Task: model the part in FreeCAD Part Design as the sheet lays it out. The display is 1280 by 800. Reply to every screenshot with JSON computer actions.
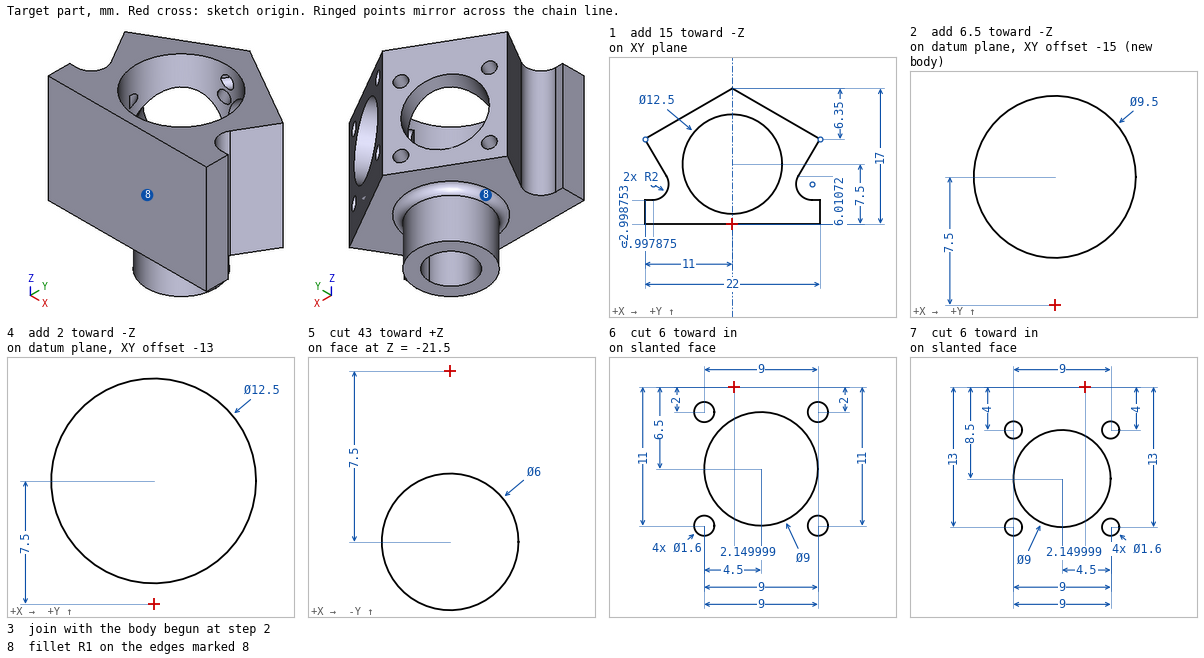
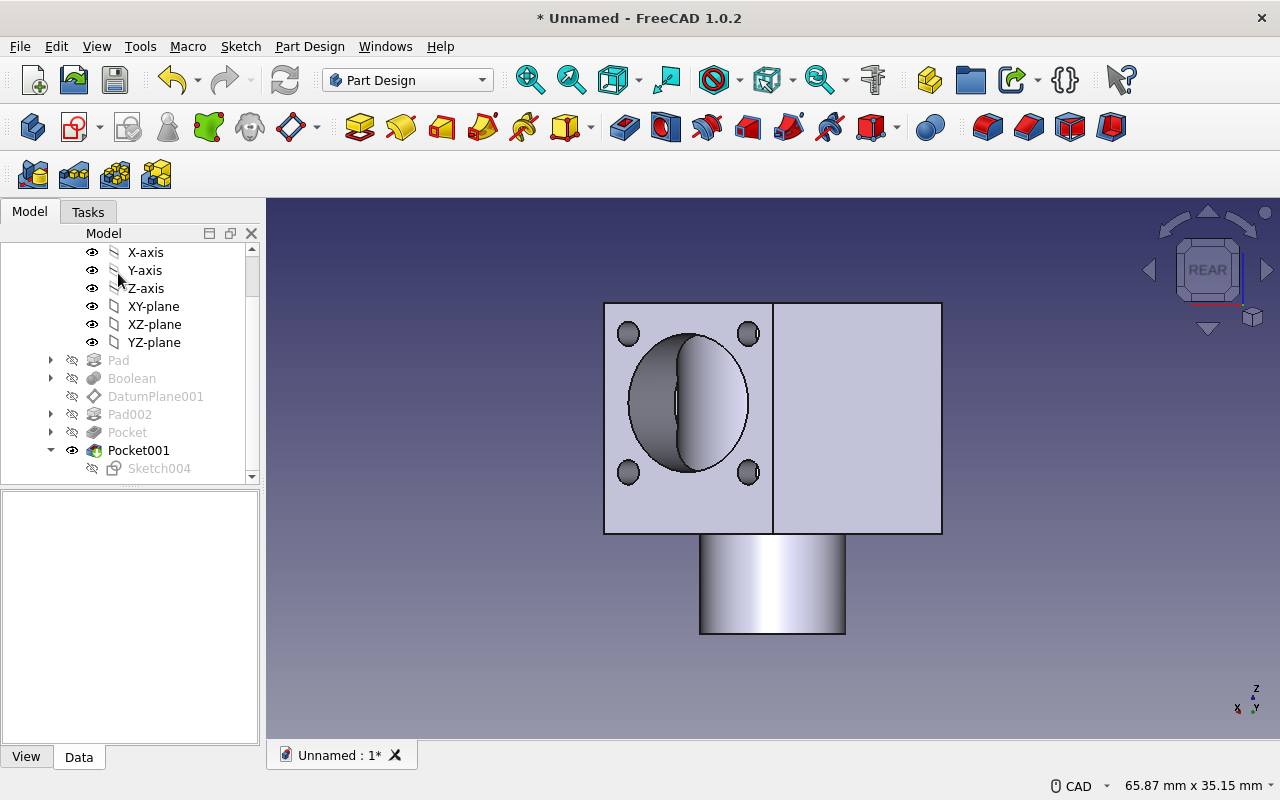
{"action": "left_click", "coordinate": [858, 417]}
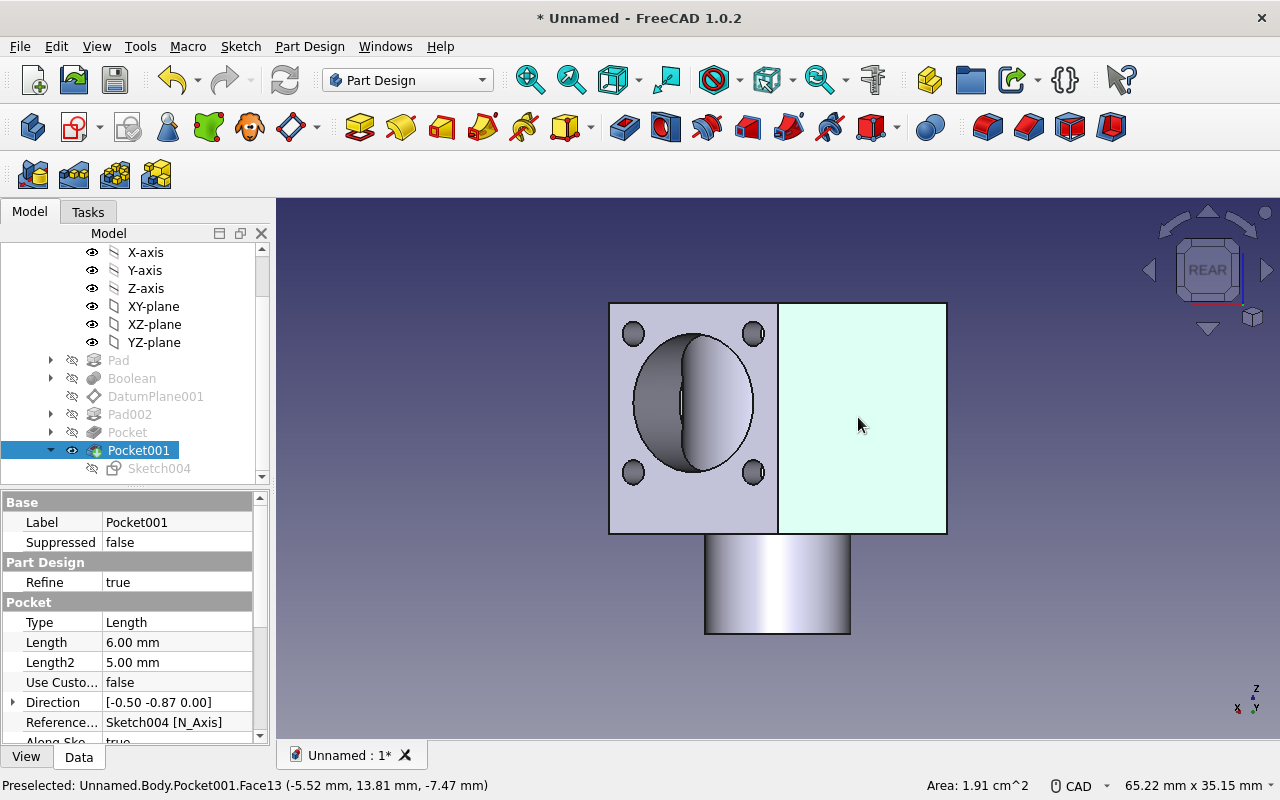
{"action": "left_click", "coordinate": [74, 128]}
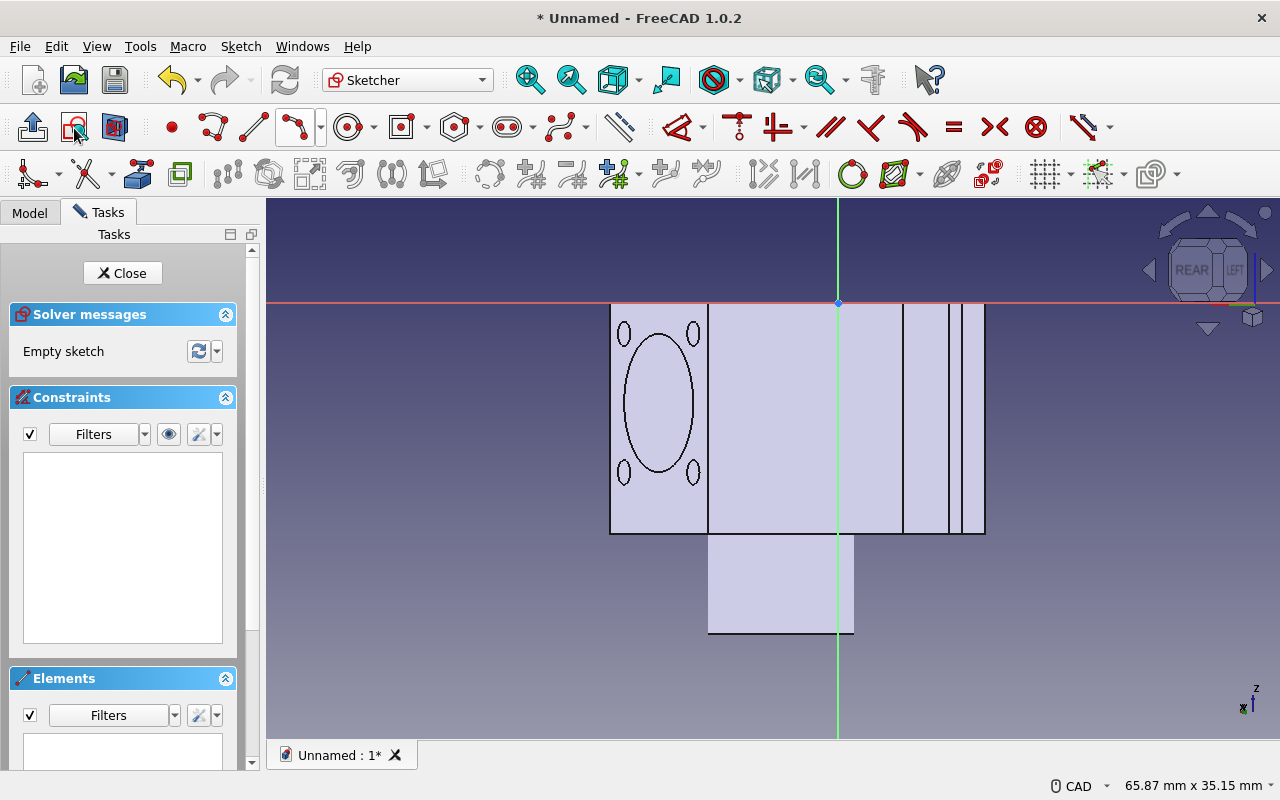
{"action": "left_click", "coordinate": [115, 128]}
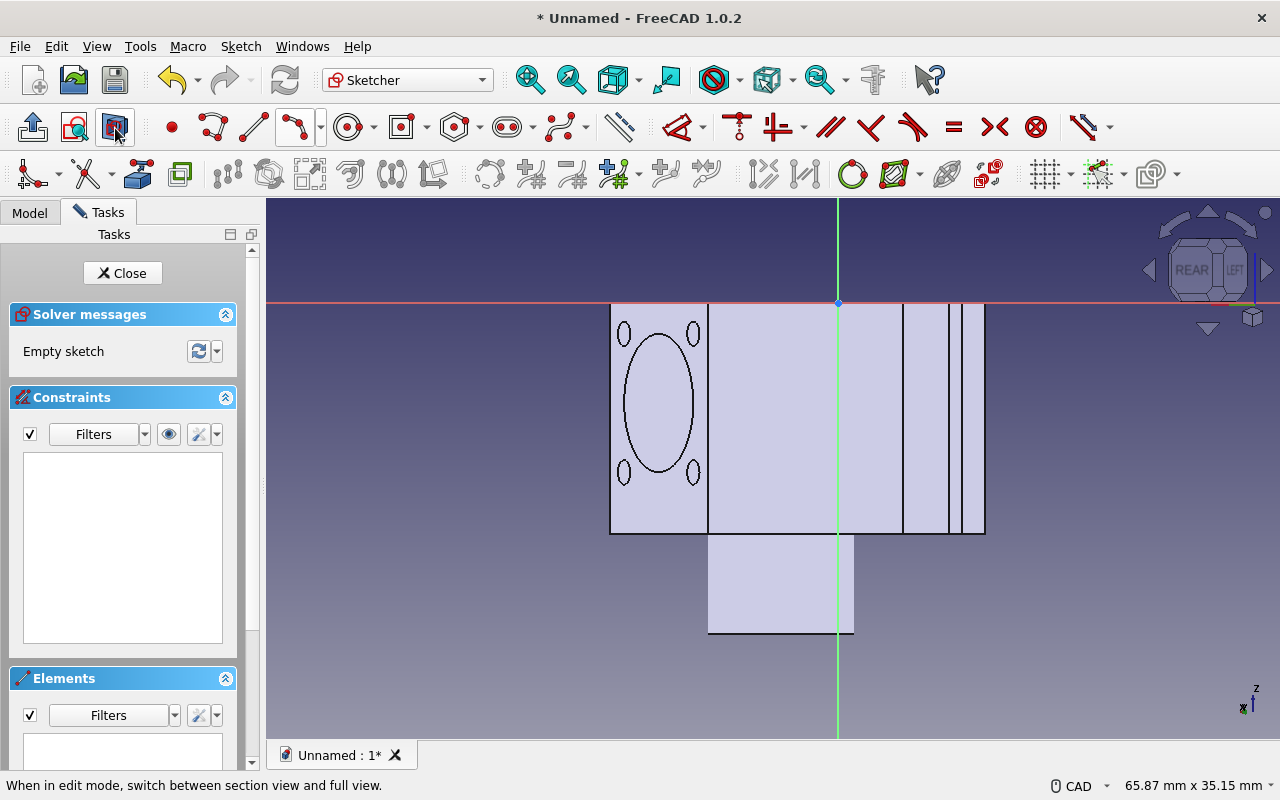
{"action": "scroll", "coordinate": [1010, 289], "scroll_direction": "up", "scroll_amount": 2}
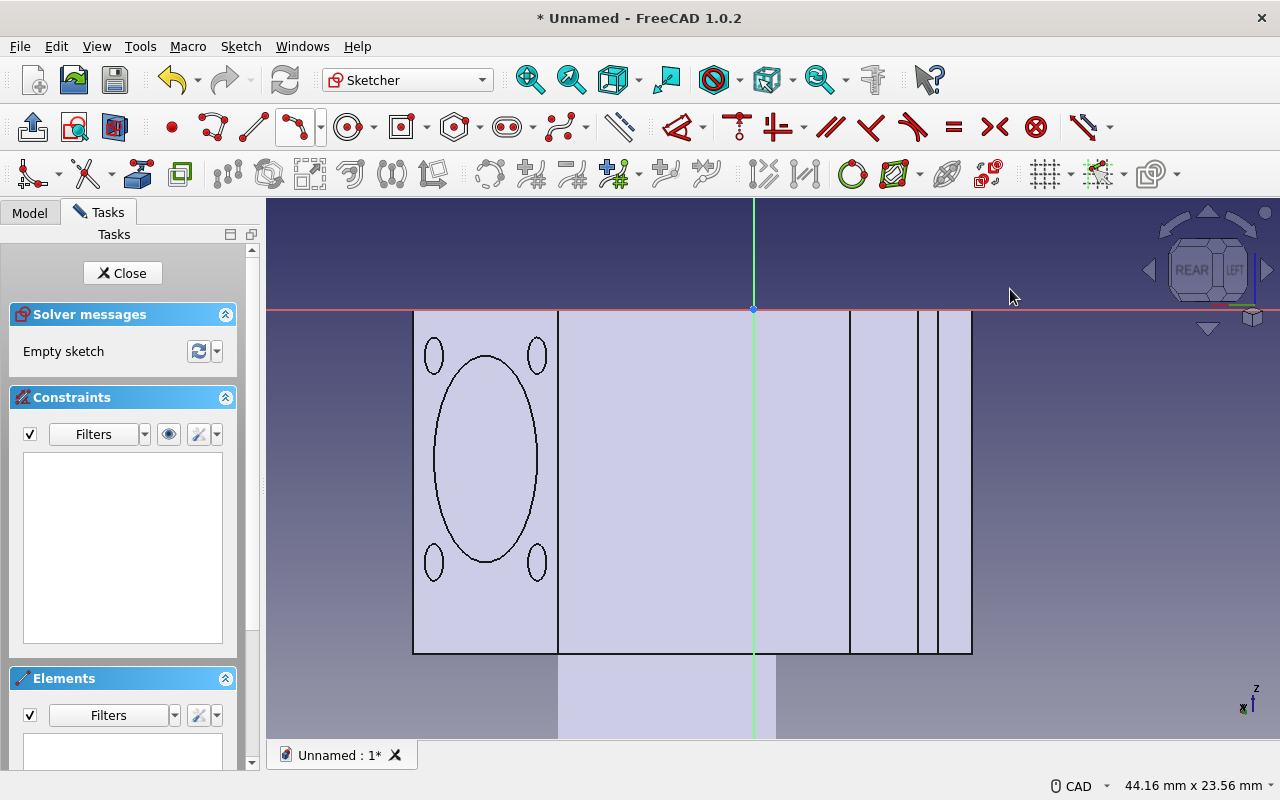
{"action": "left_click", "coordinate": [348, 128]}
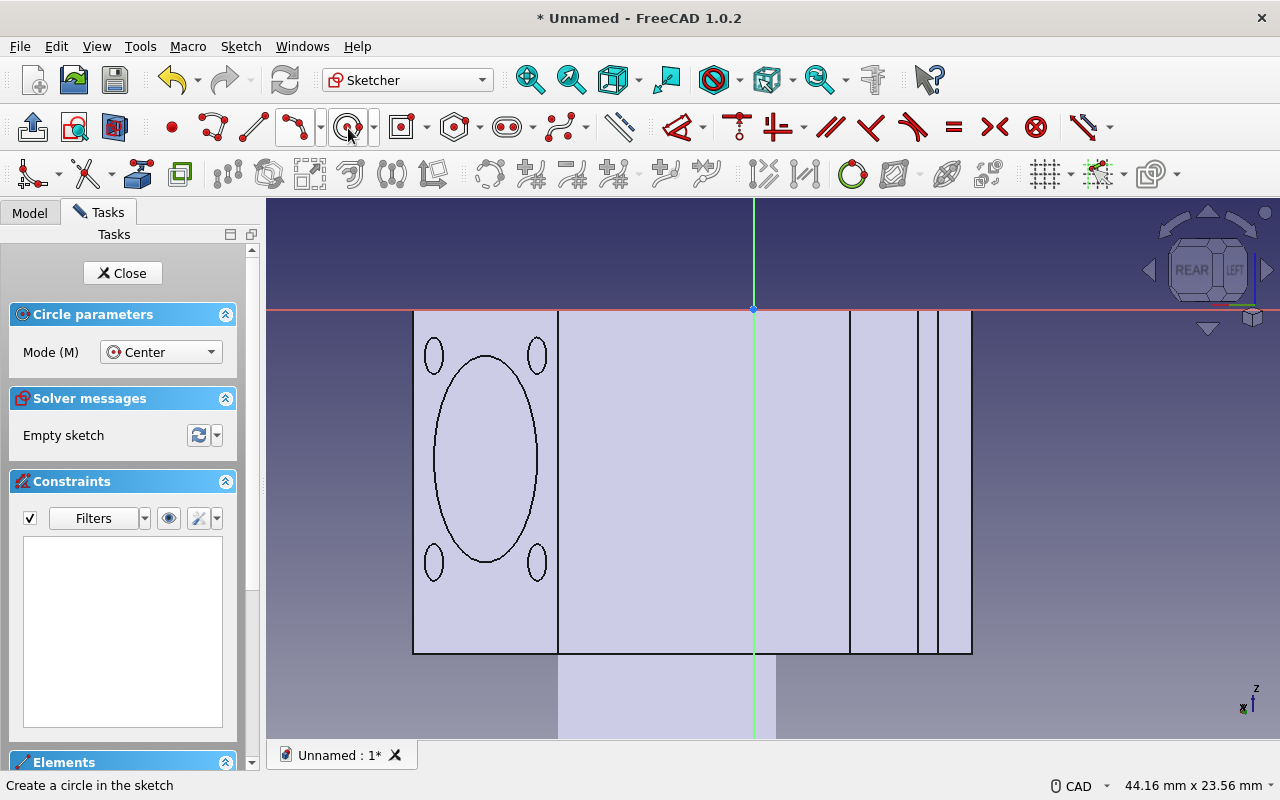
{"action": "left_click", "coordinate": [704, 505]}
{"action": "mouse_move", "coordinate": [777, 432]}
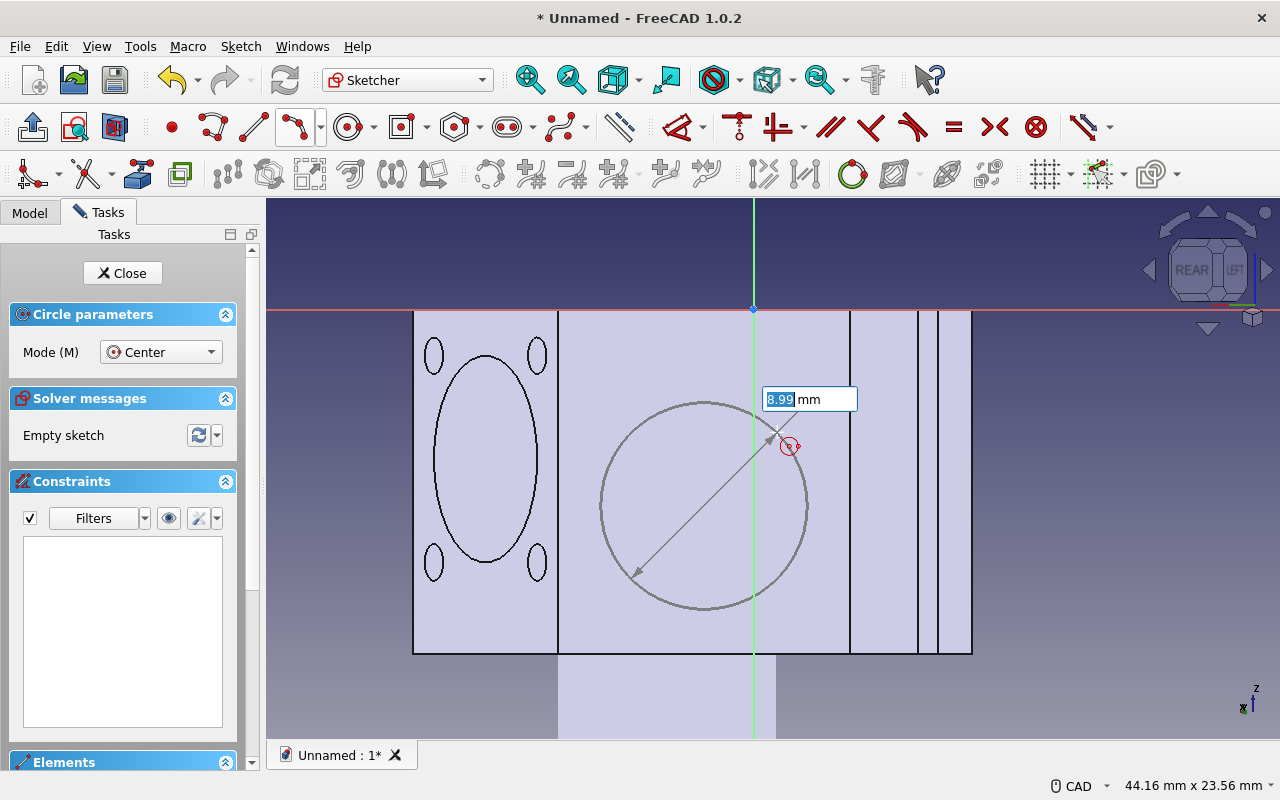
{"action": "type", "text": "9"}
{"action": "key", "text": "Return"}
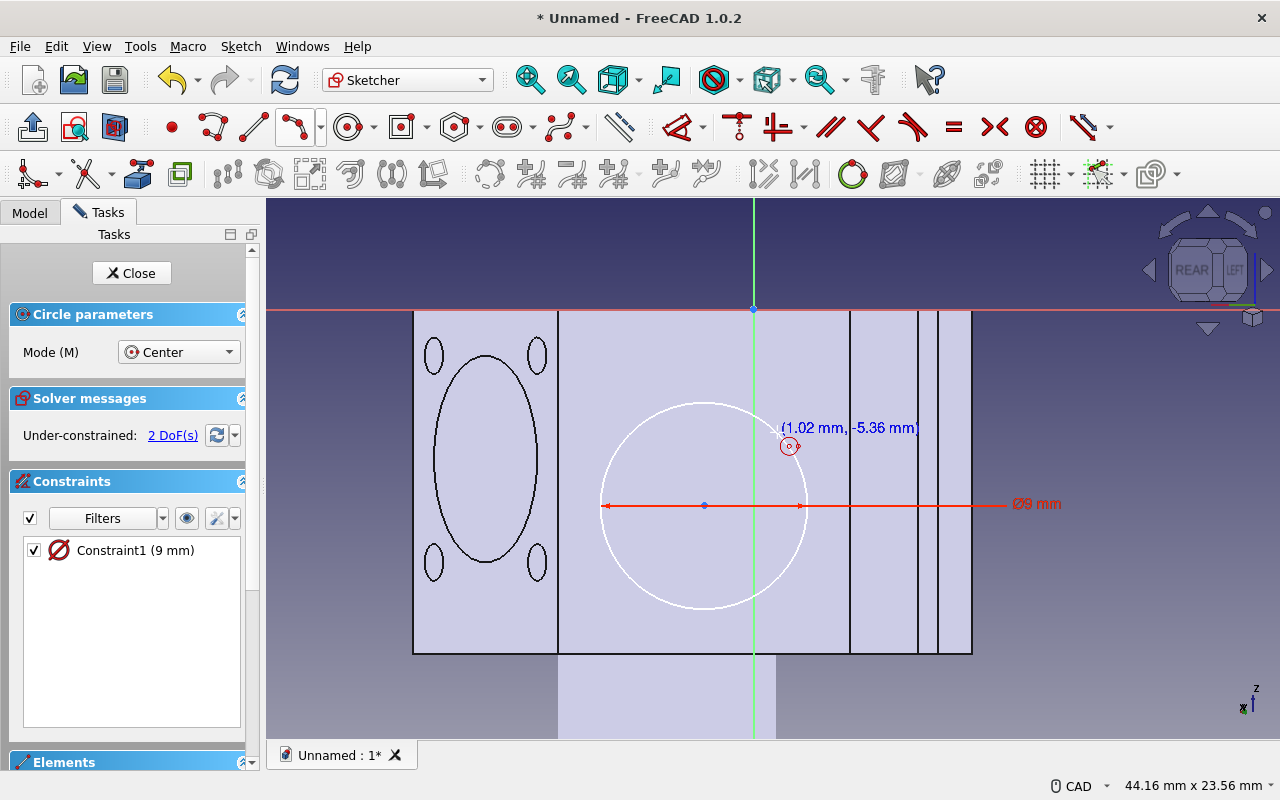
{"action": "scroll", "coordinate": [808, 608], "scroll_direction": "up", "scroll_amount": 2}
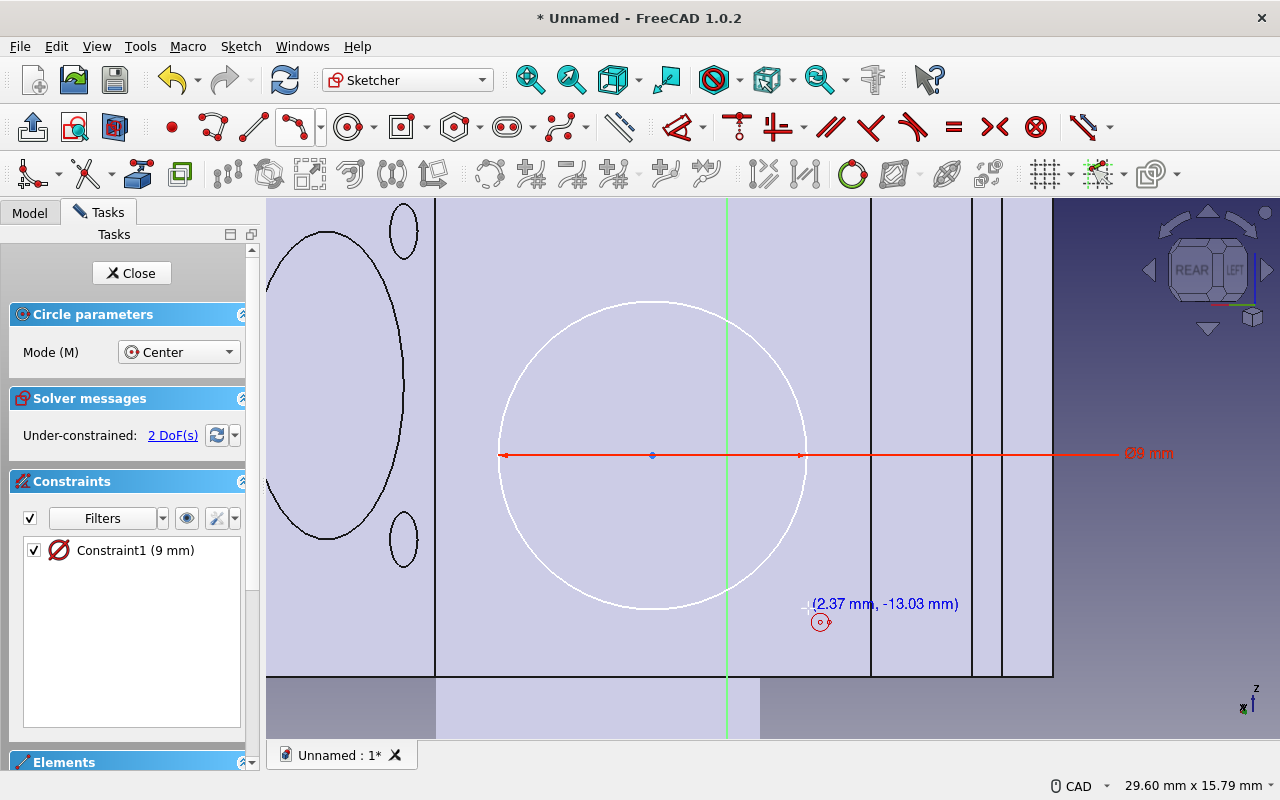
{"action": "left_click", "coordinate": [807, 608]}
{"action": "mouse_move", "coordinate": [827, 589]}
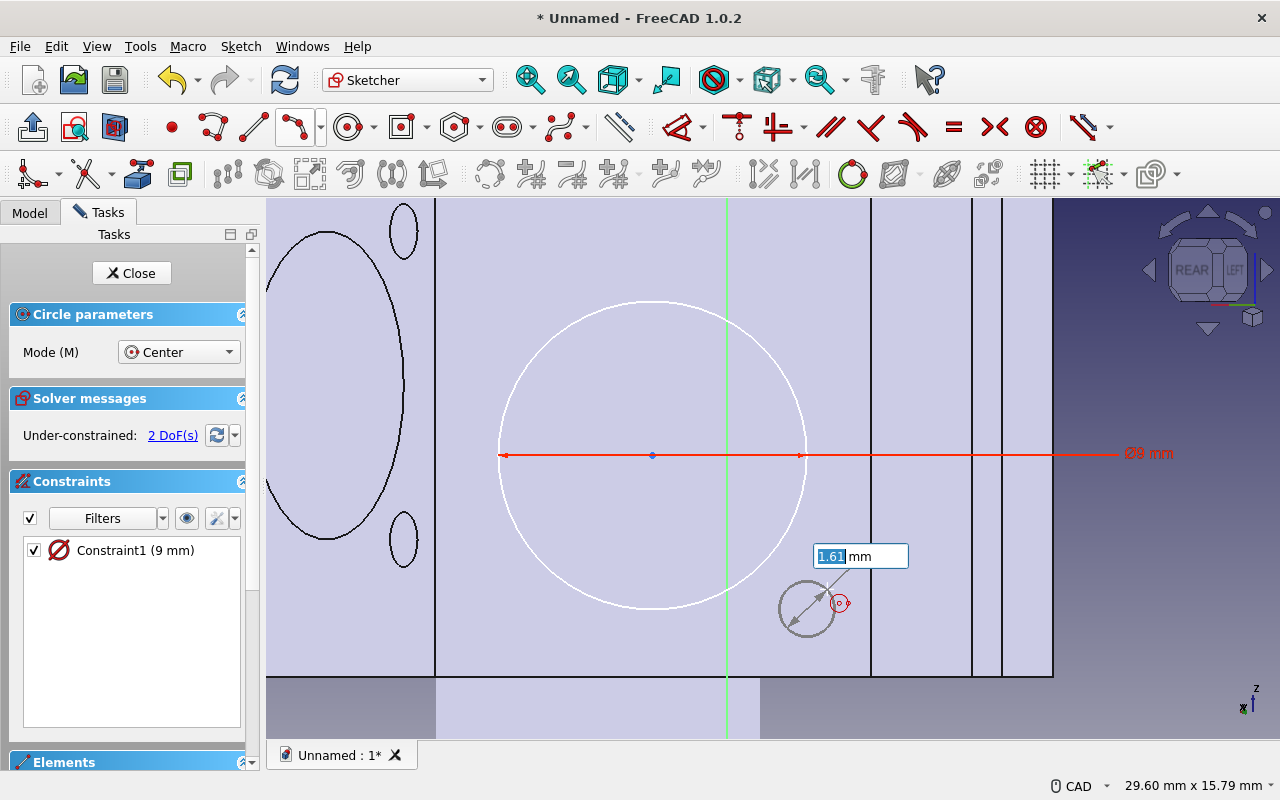
{"action": "type", "text": "1.6"}
{"action": "key", "text": "Return"}